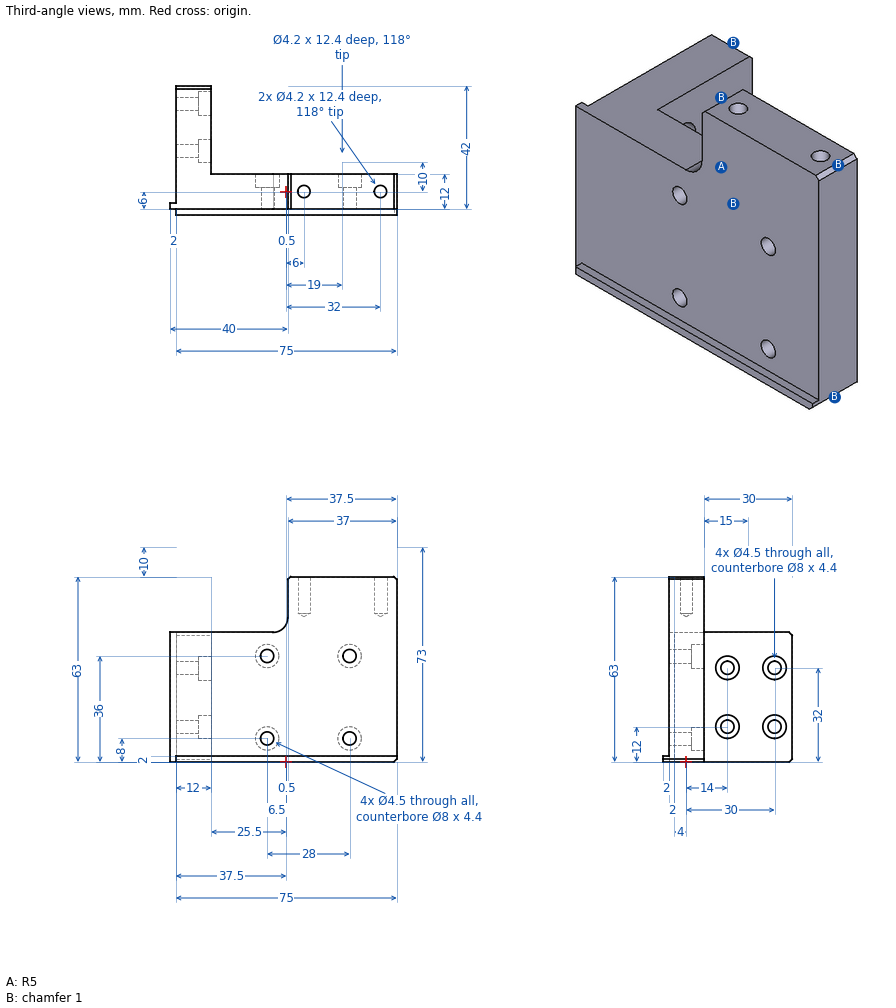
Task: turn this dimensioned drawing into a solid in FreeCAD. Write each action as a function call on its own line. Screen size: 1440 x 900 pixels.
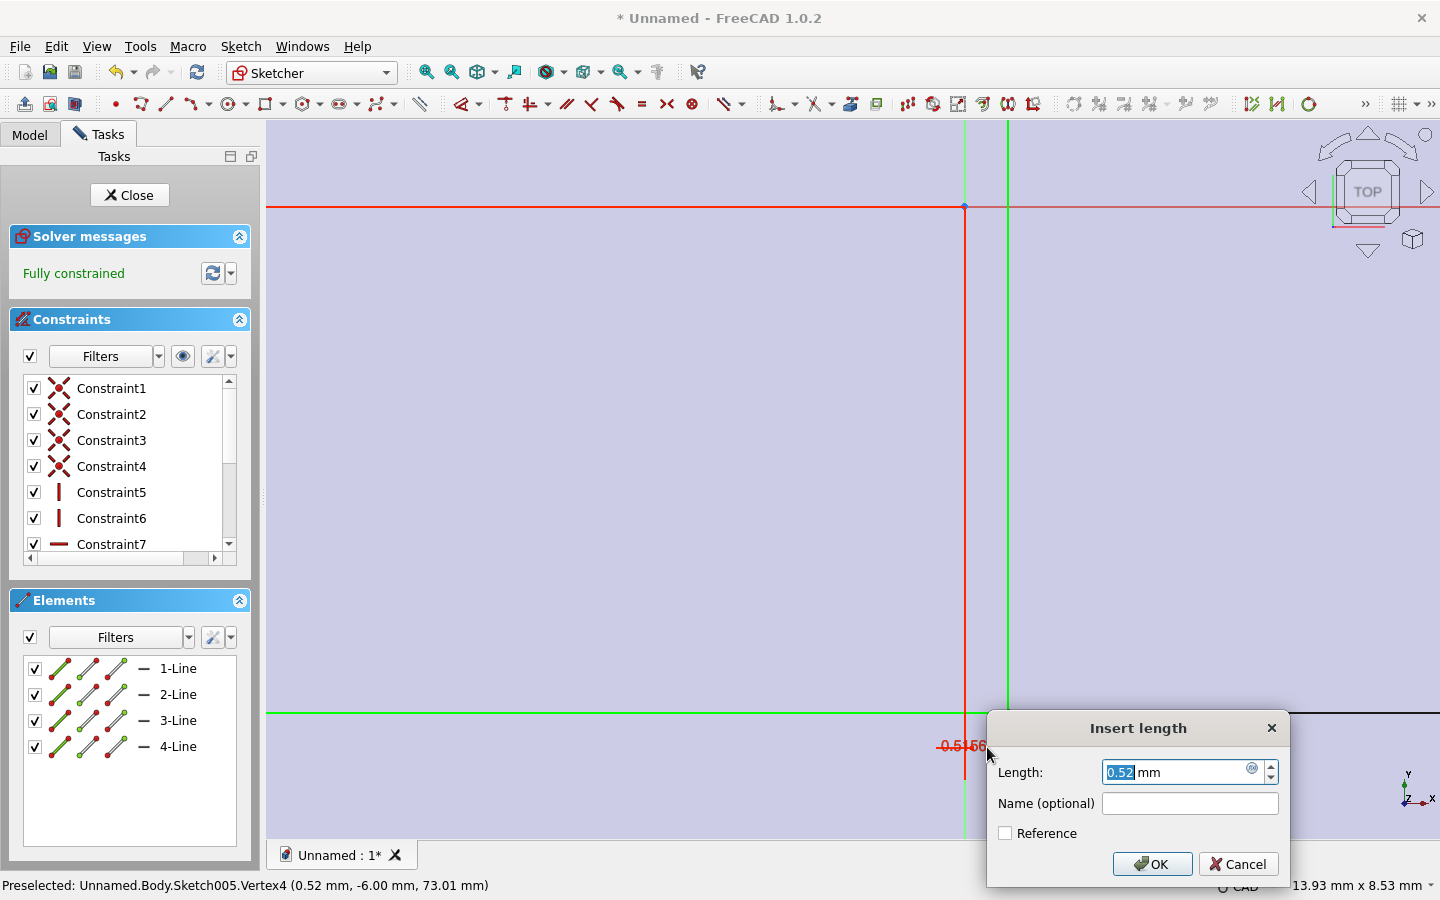
text(0.5)
key(Return)
key(Escape)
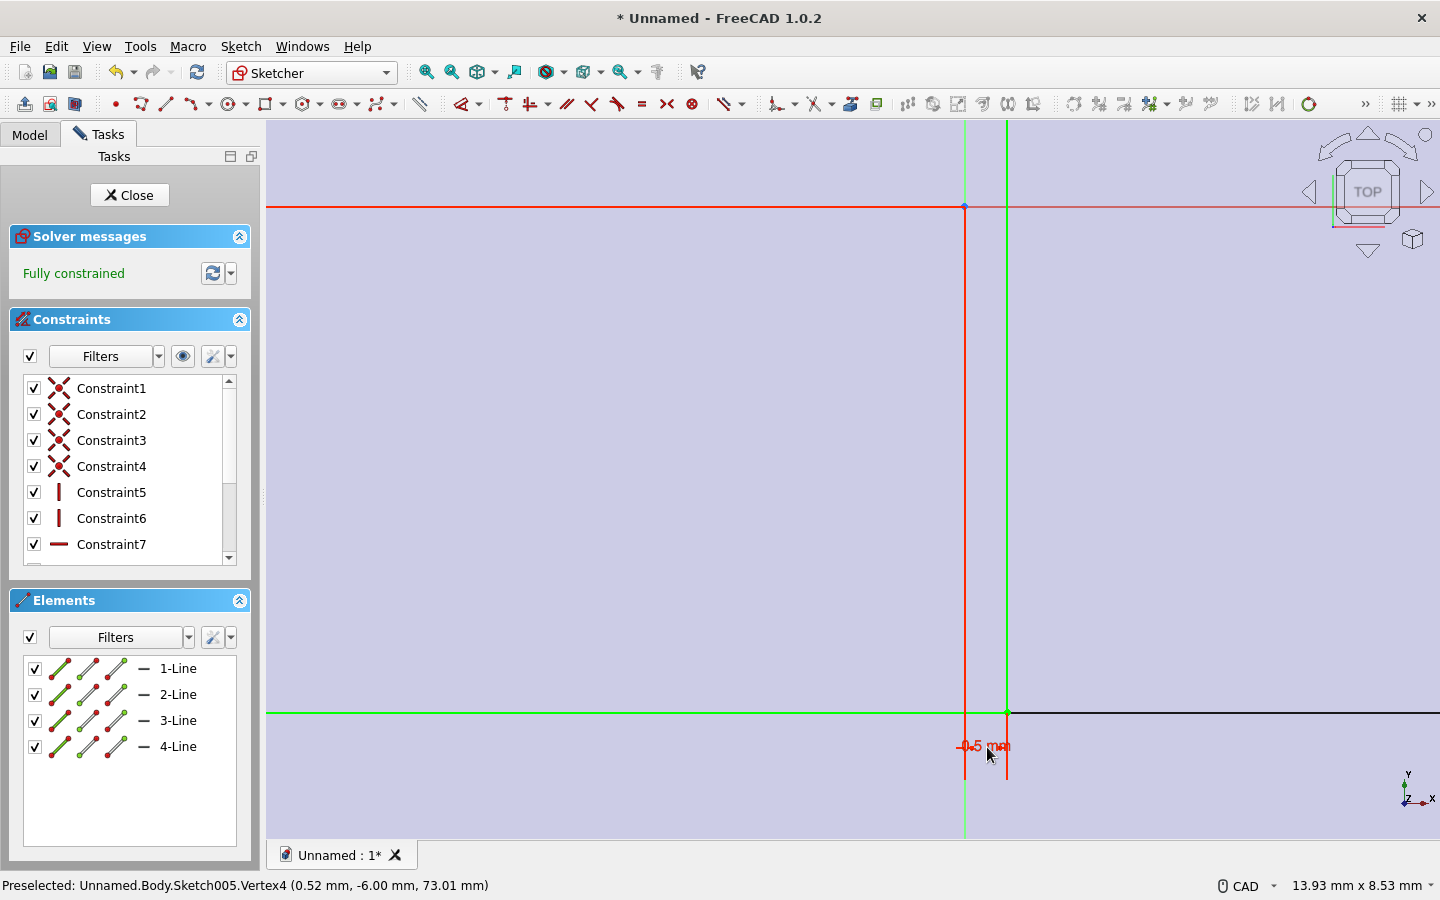
click(130, 195)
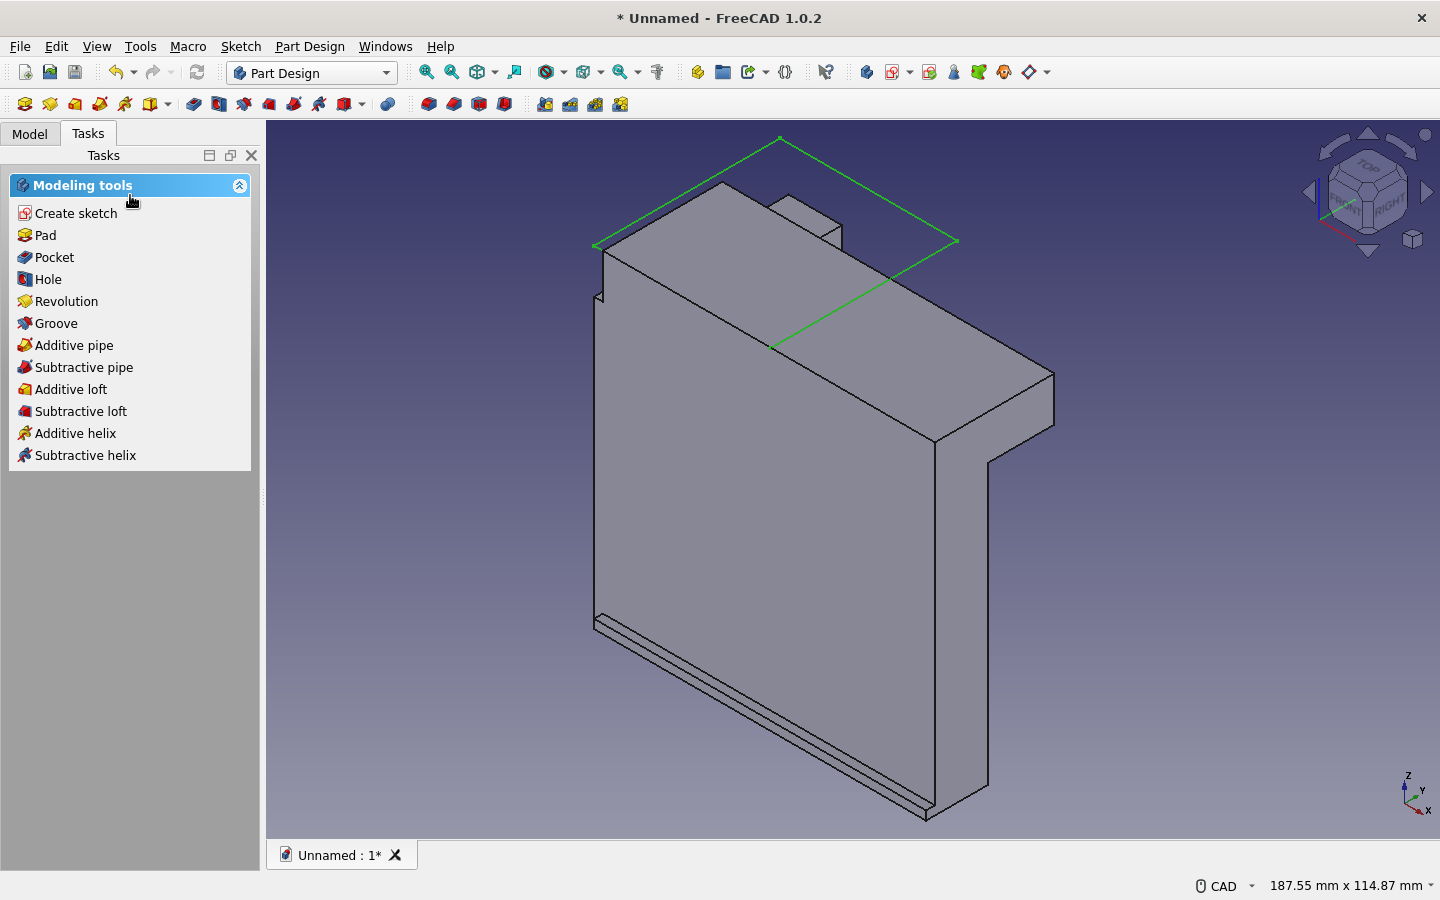
click(194, 104)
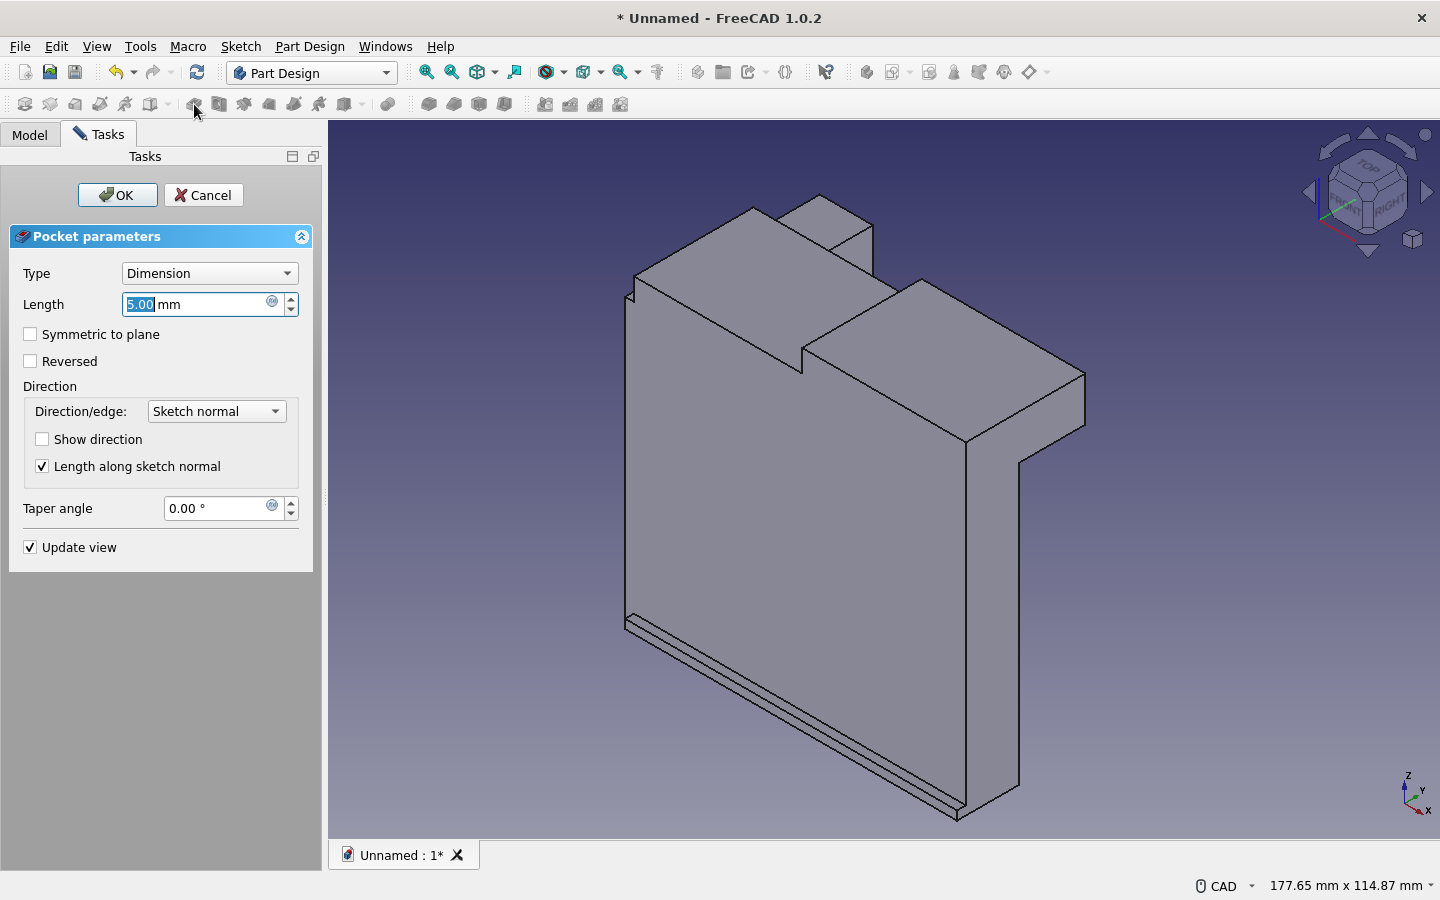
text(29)
key(Tab)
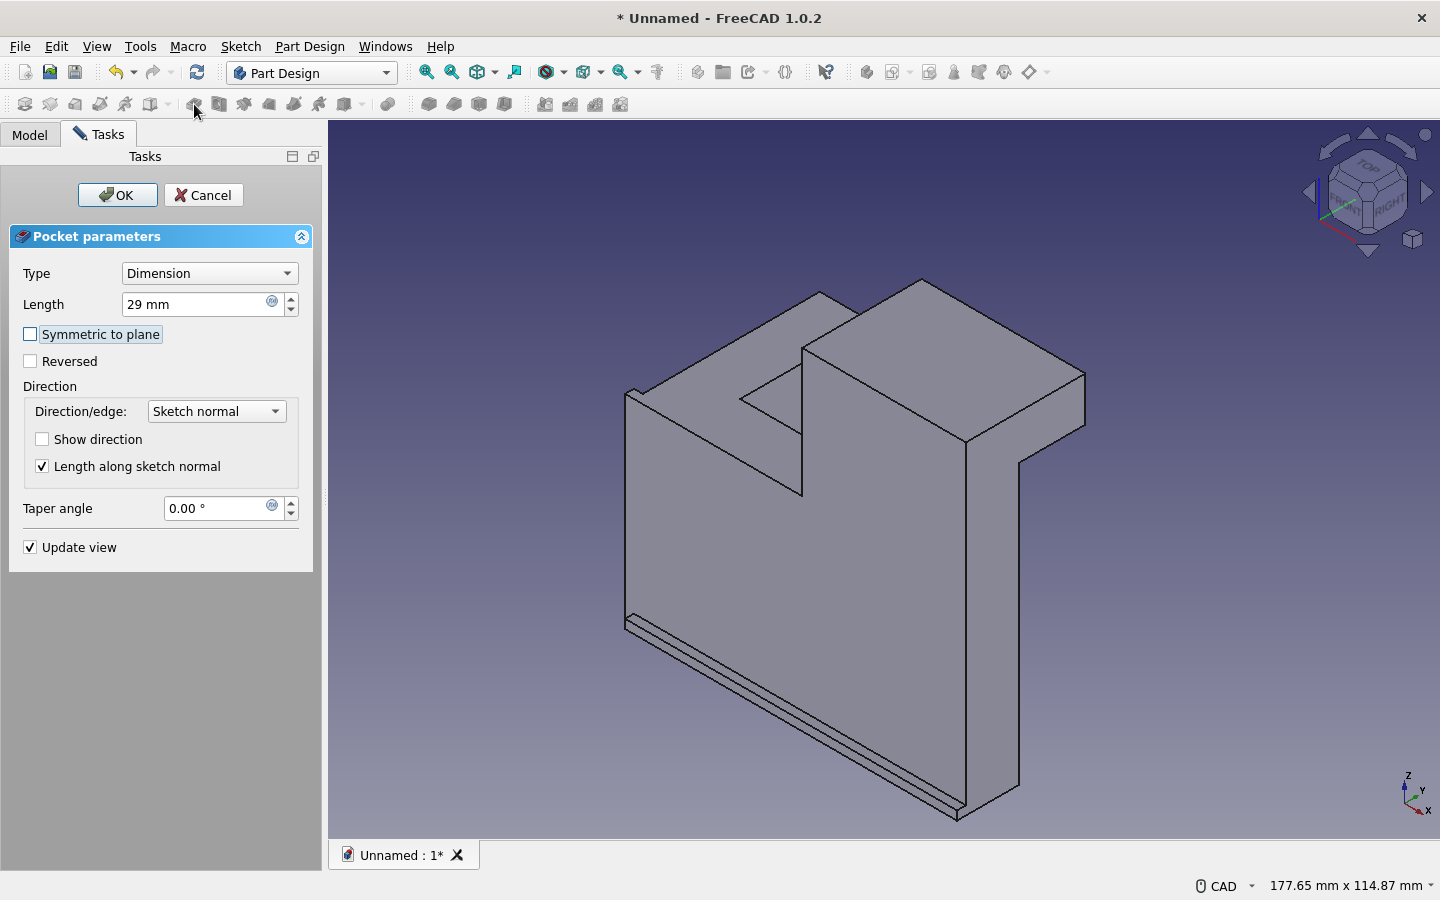
click(118, 195)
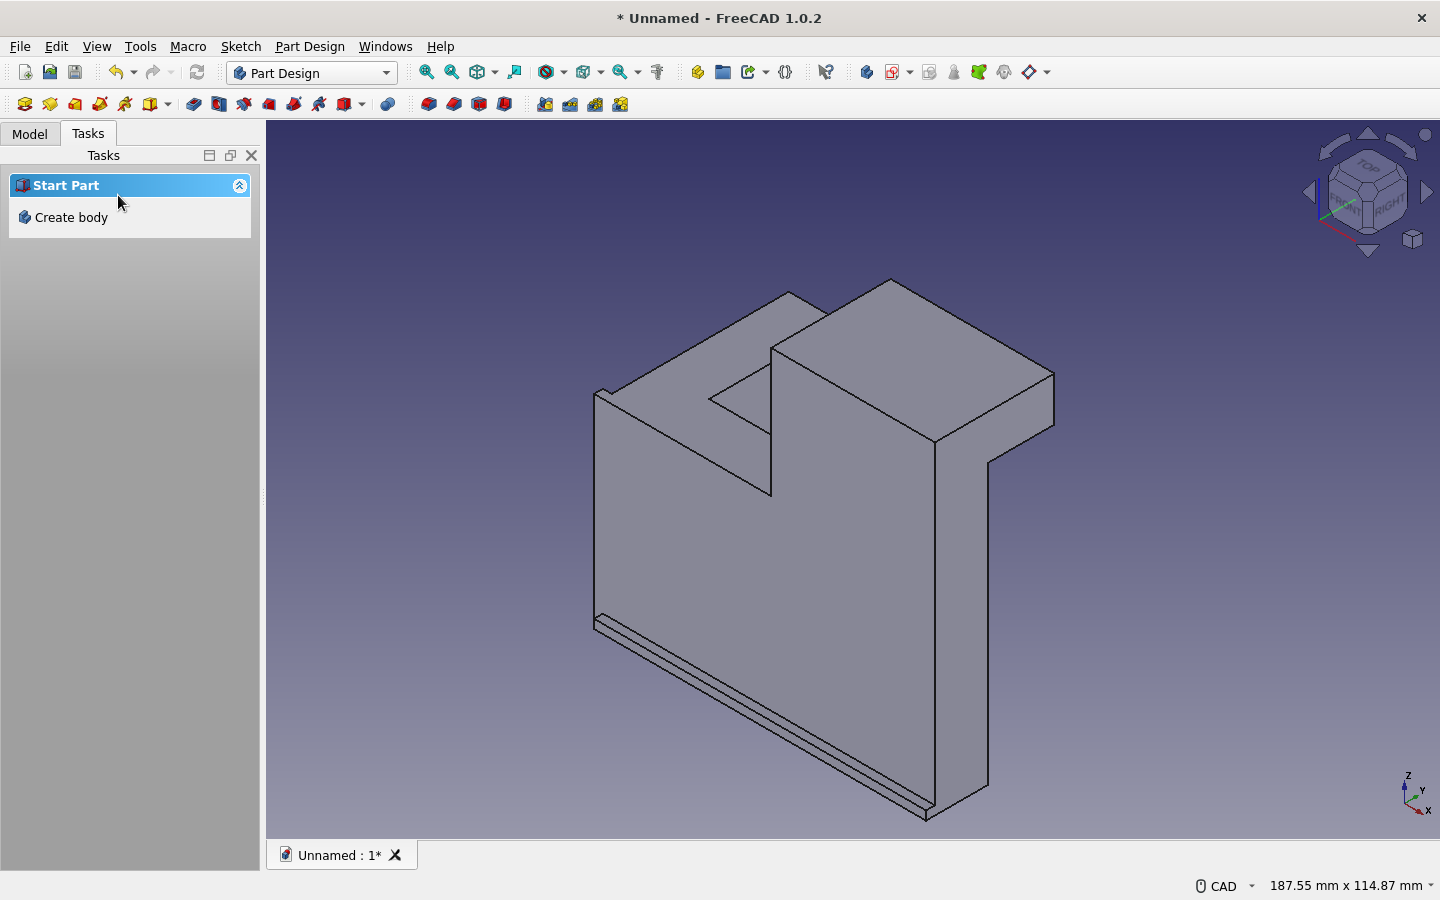
click(913, 360)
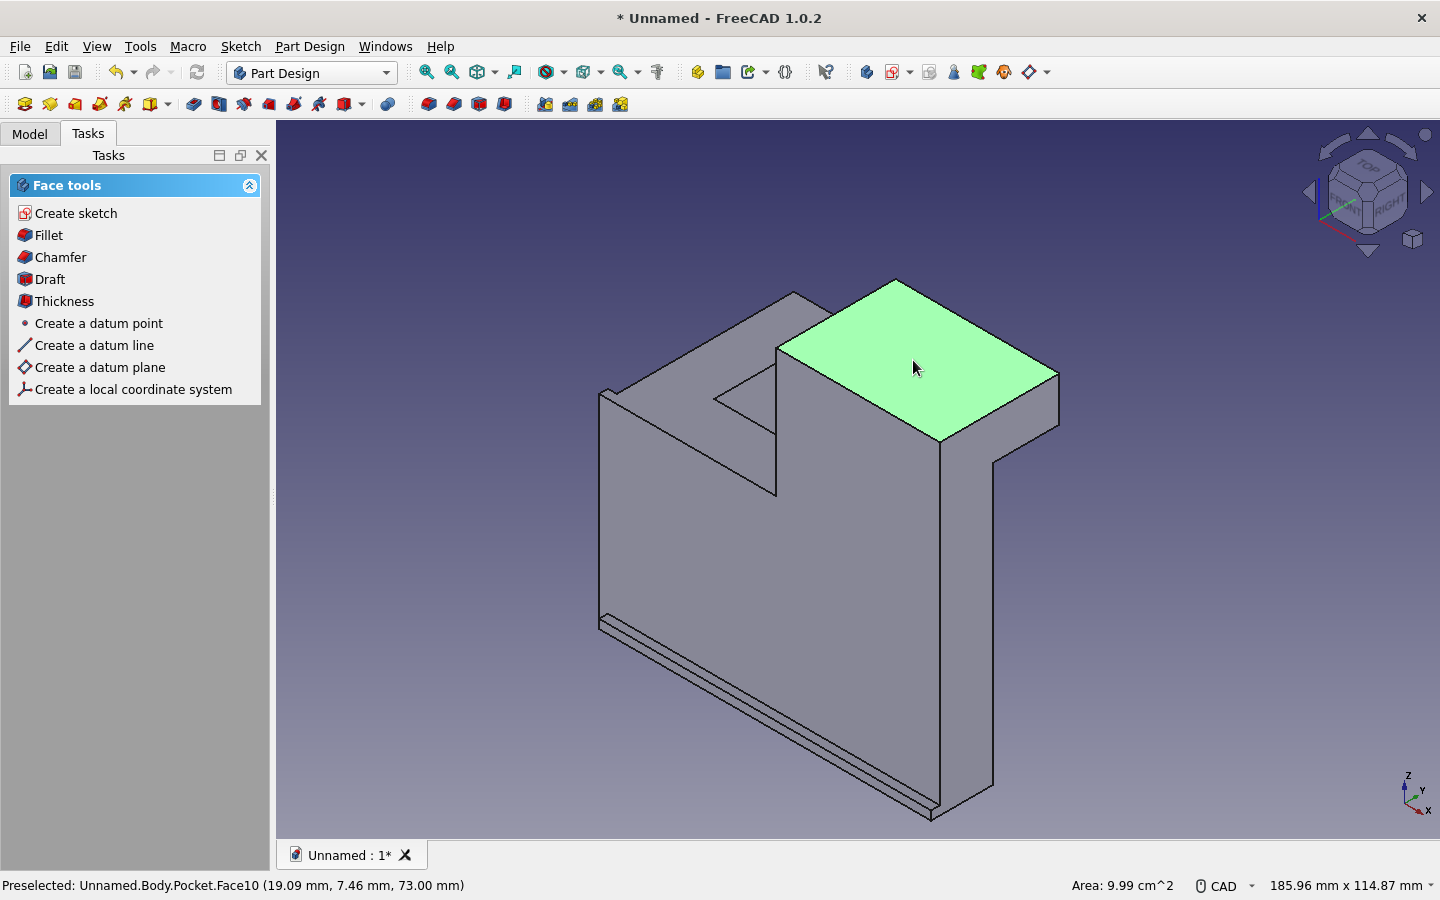
click(892, 72)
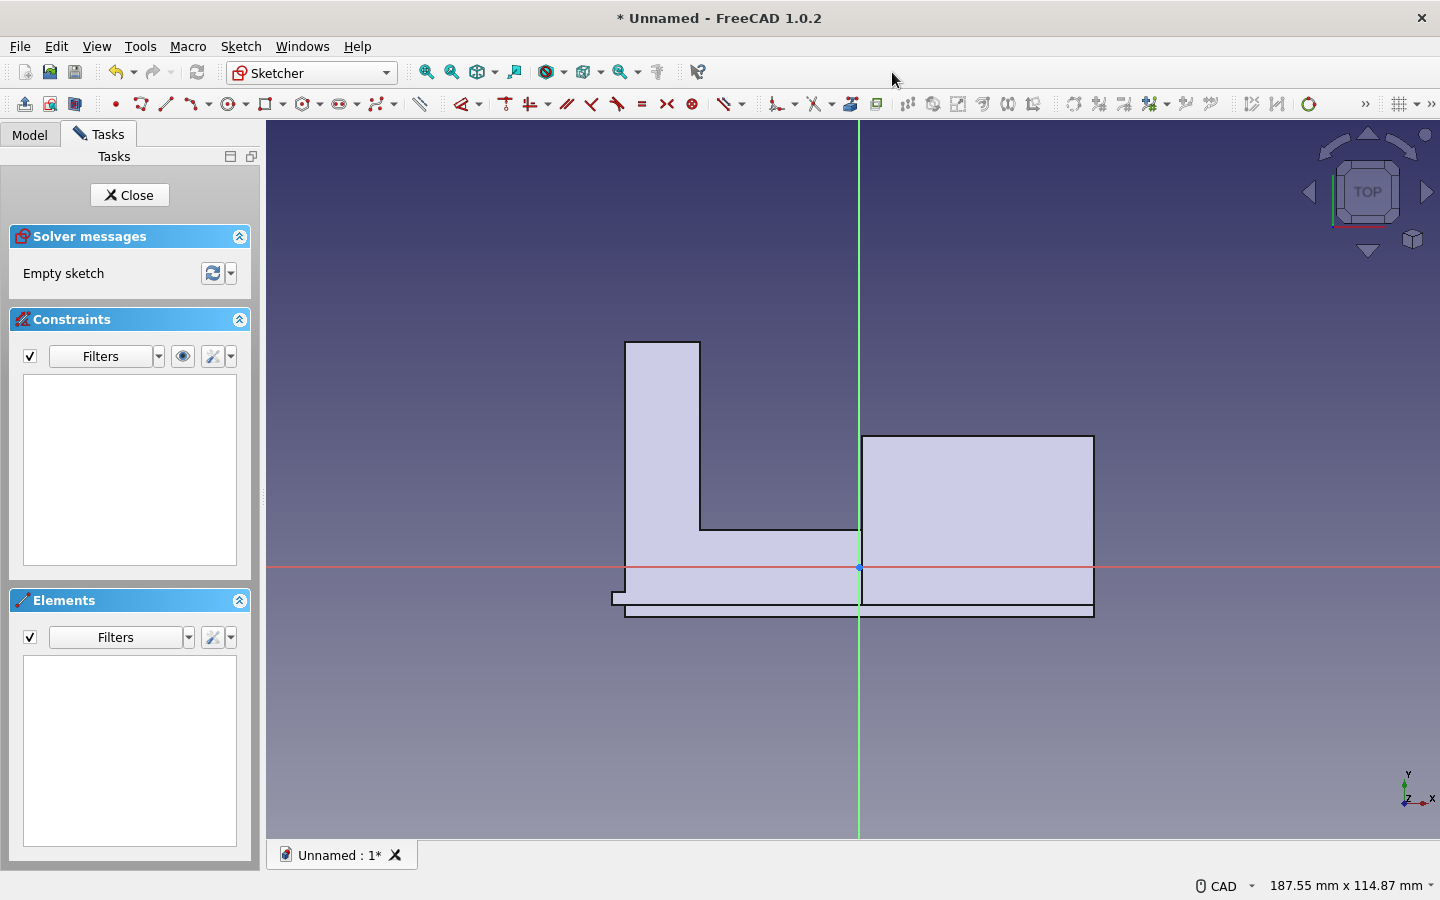
scroll(991, 506, up, 14)